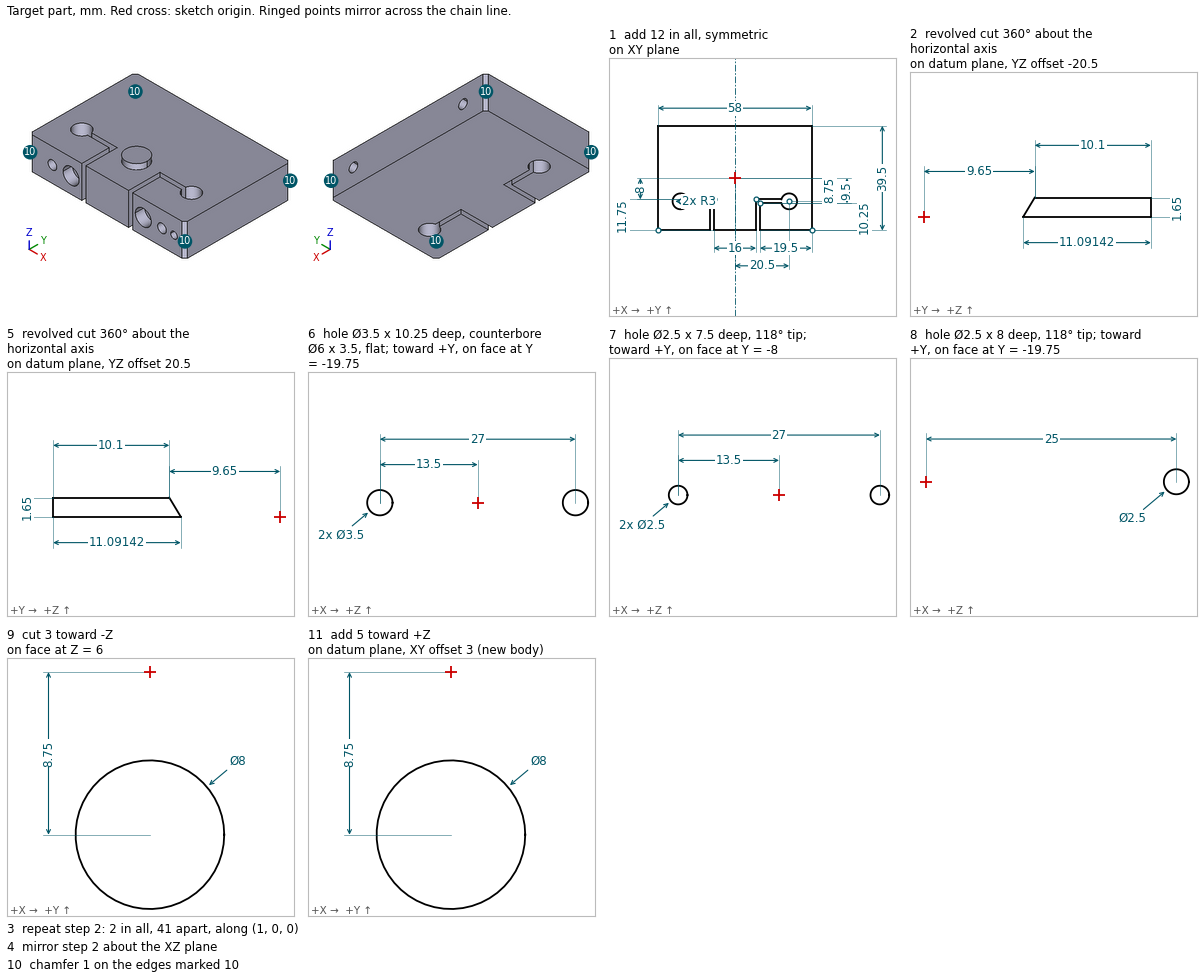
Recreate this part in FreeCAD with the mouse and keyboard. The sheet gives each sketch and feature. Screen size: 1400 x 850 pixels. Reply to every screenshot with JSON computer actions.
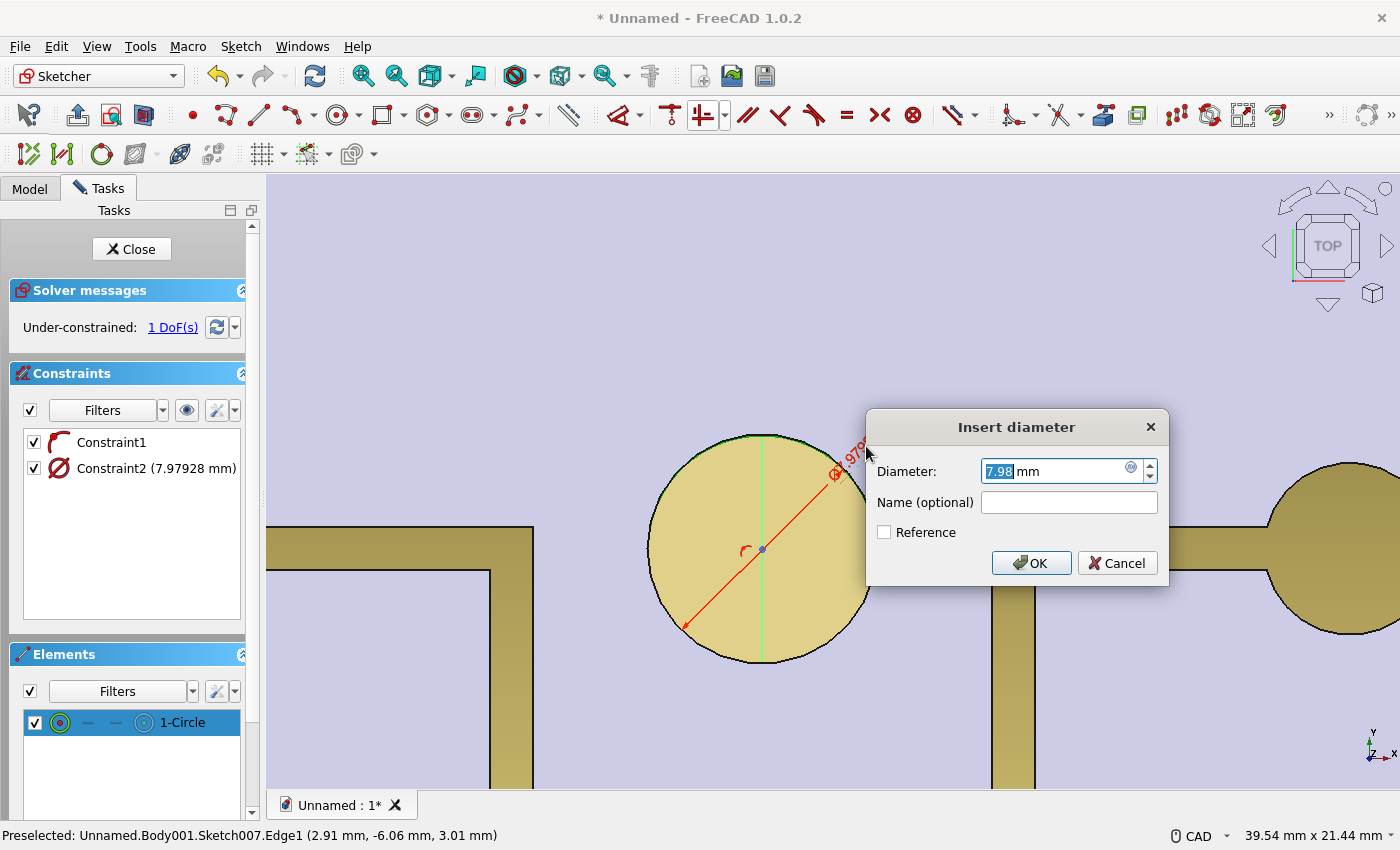
{"action": "type", "text": "8"}
{"action": "key", "text": "Return"}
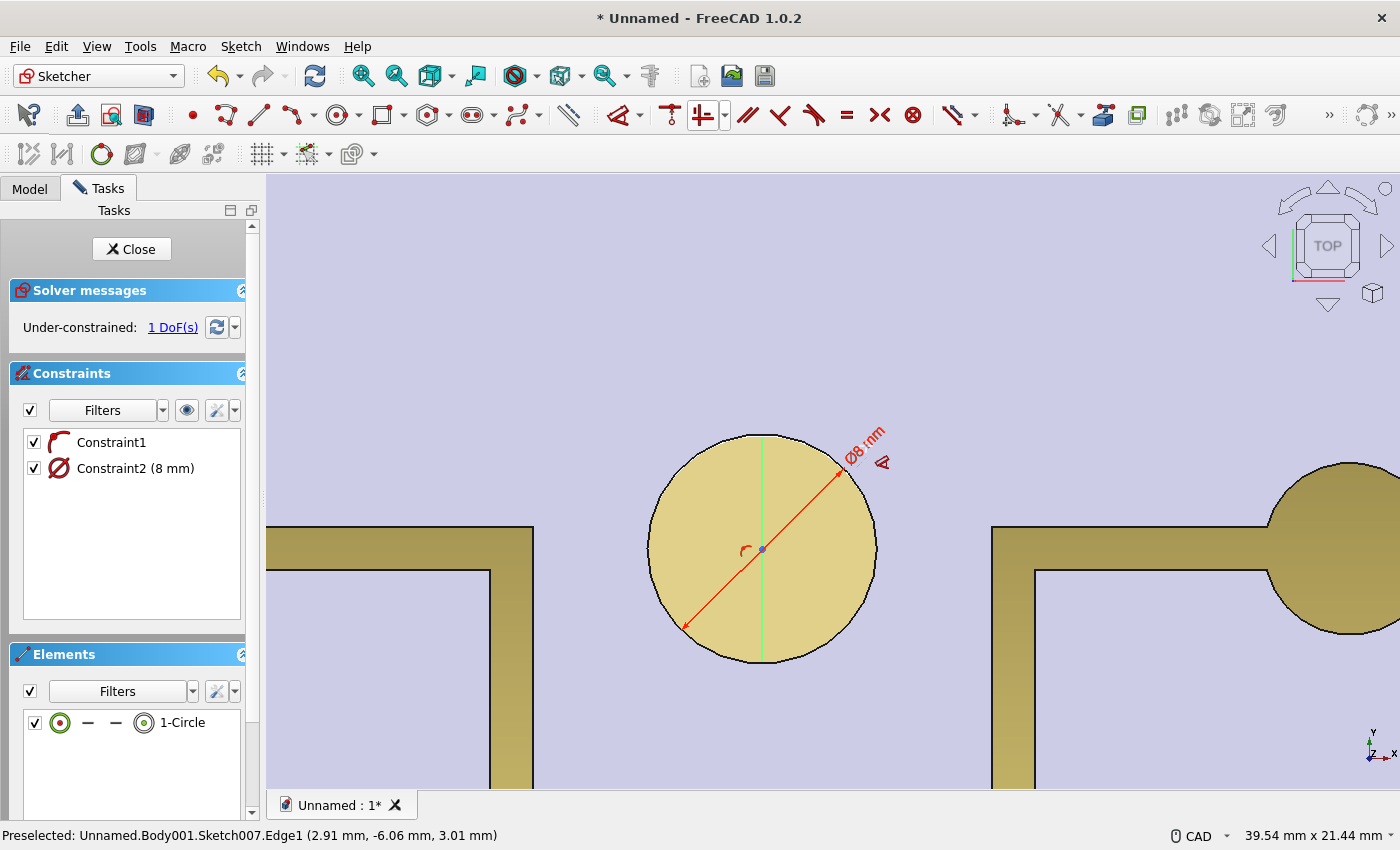
{"action": "left_click", "coordinate": [762, 550]}
{"action": "left_click", "coordinate": [796, 424]}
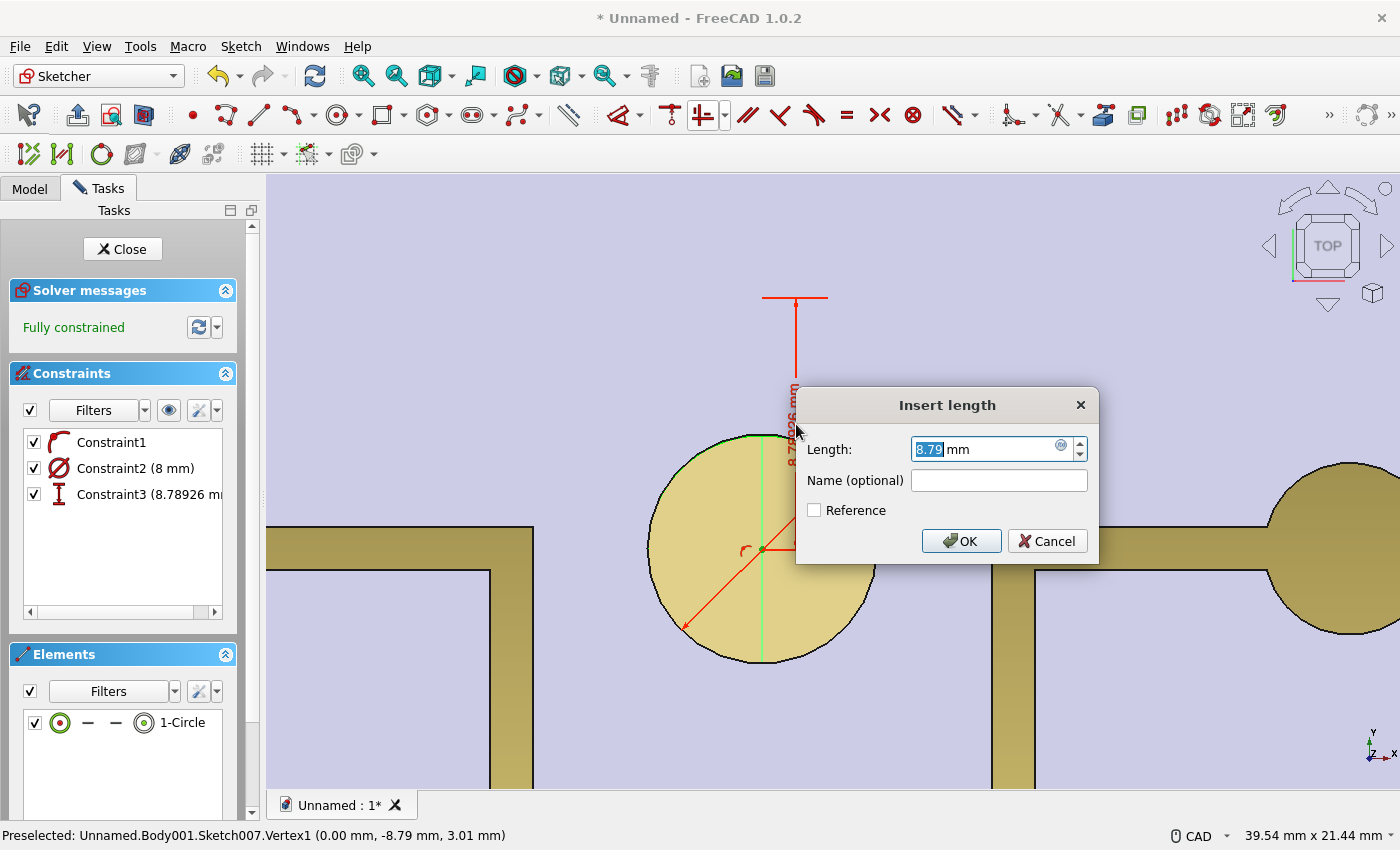
{"action": "type", "text": "8.75"}
{"action": "key", "text": "Return"}
{"action": "key", "text": "Escape"}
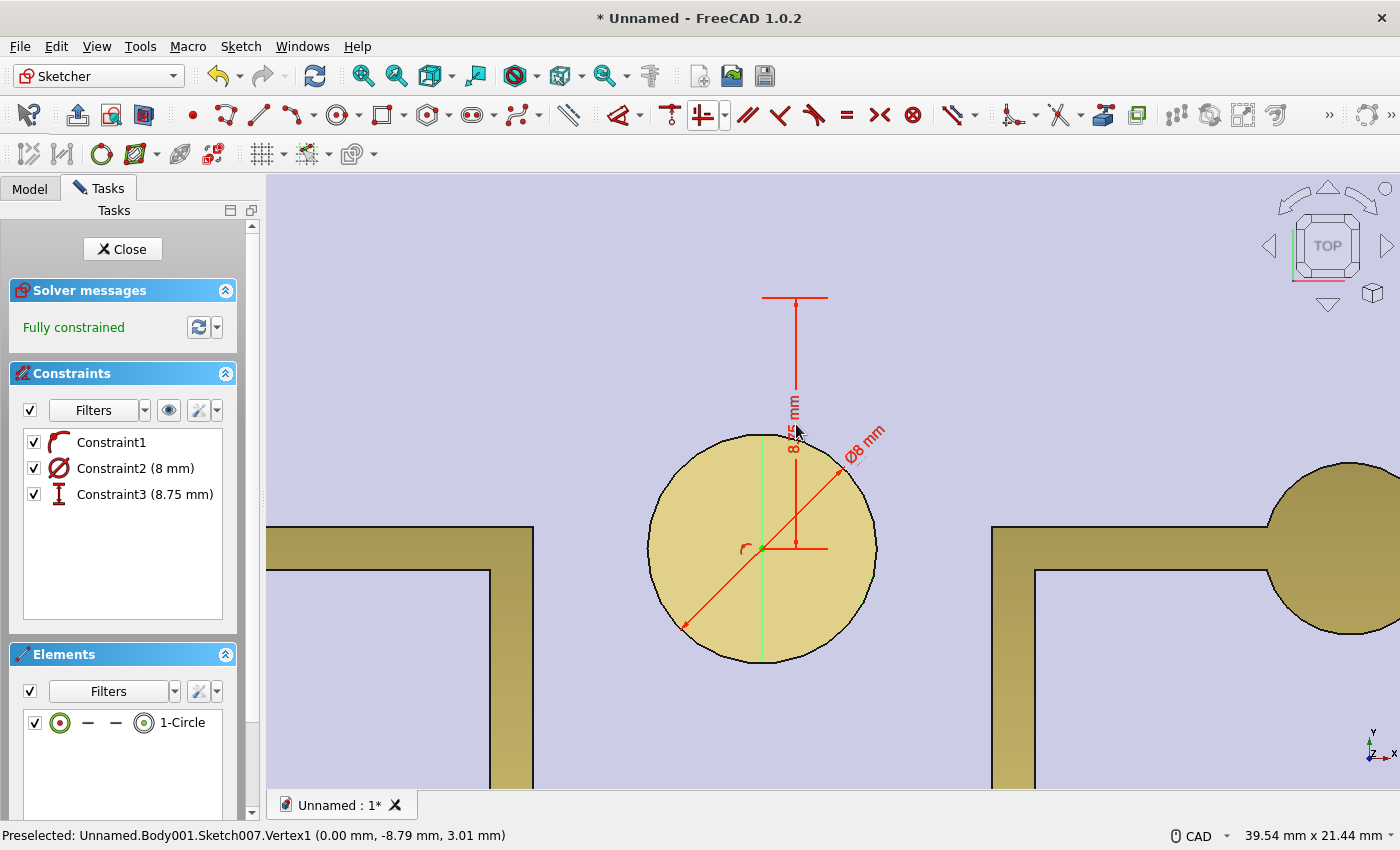
{"action": "left_click", "coordinate": [123, 249]}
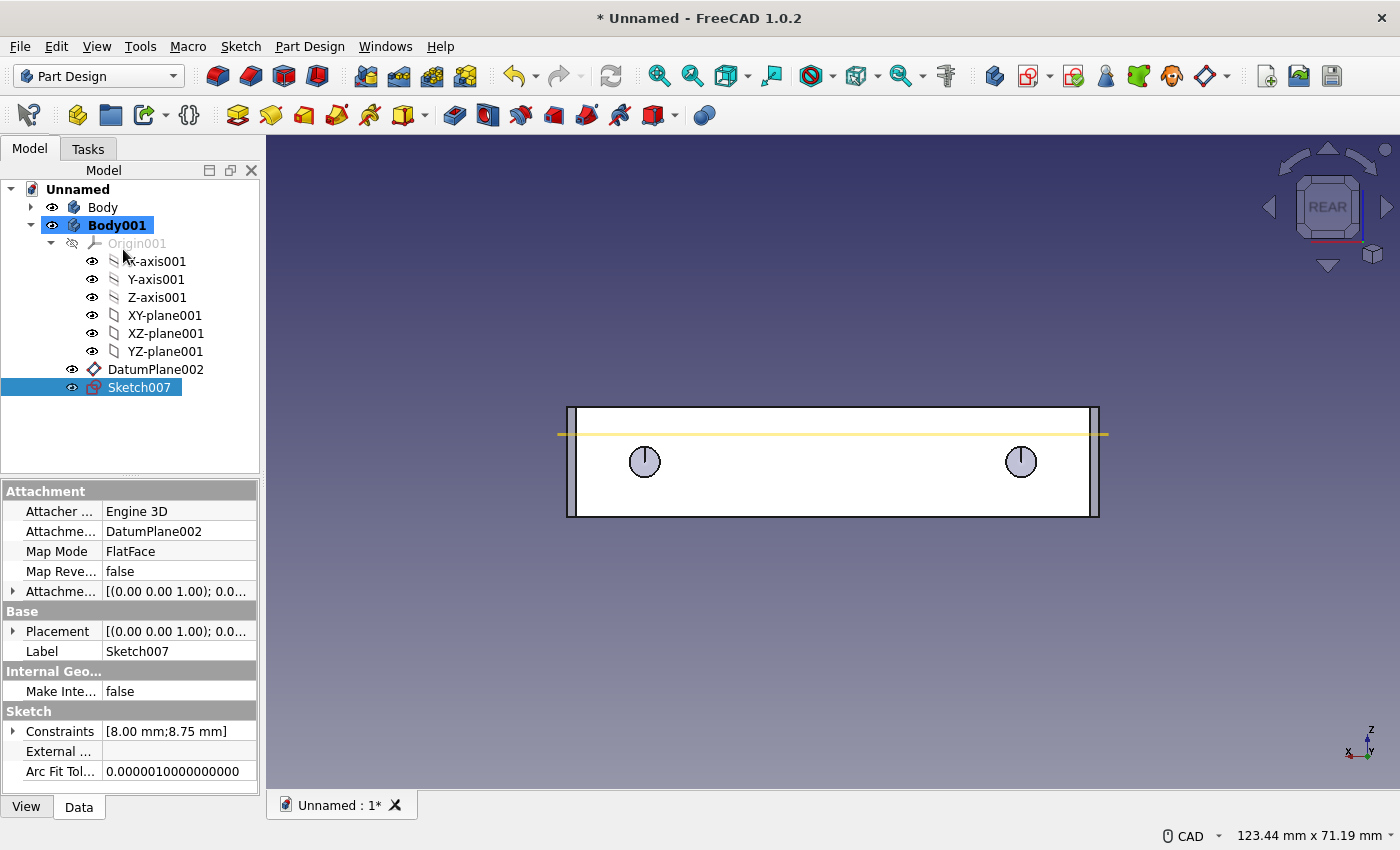
{"action": "left_click", "coordinate": [238, 116]}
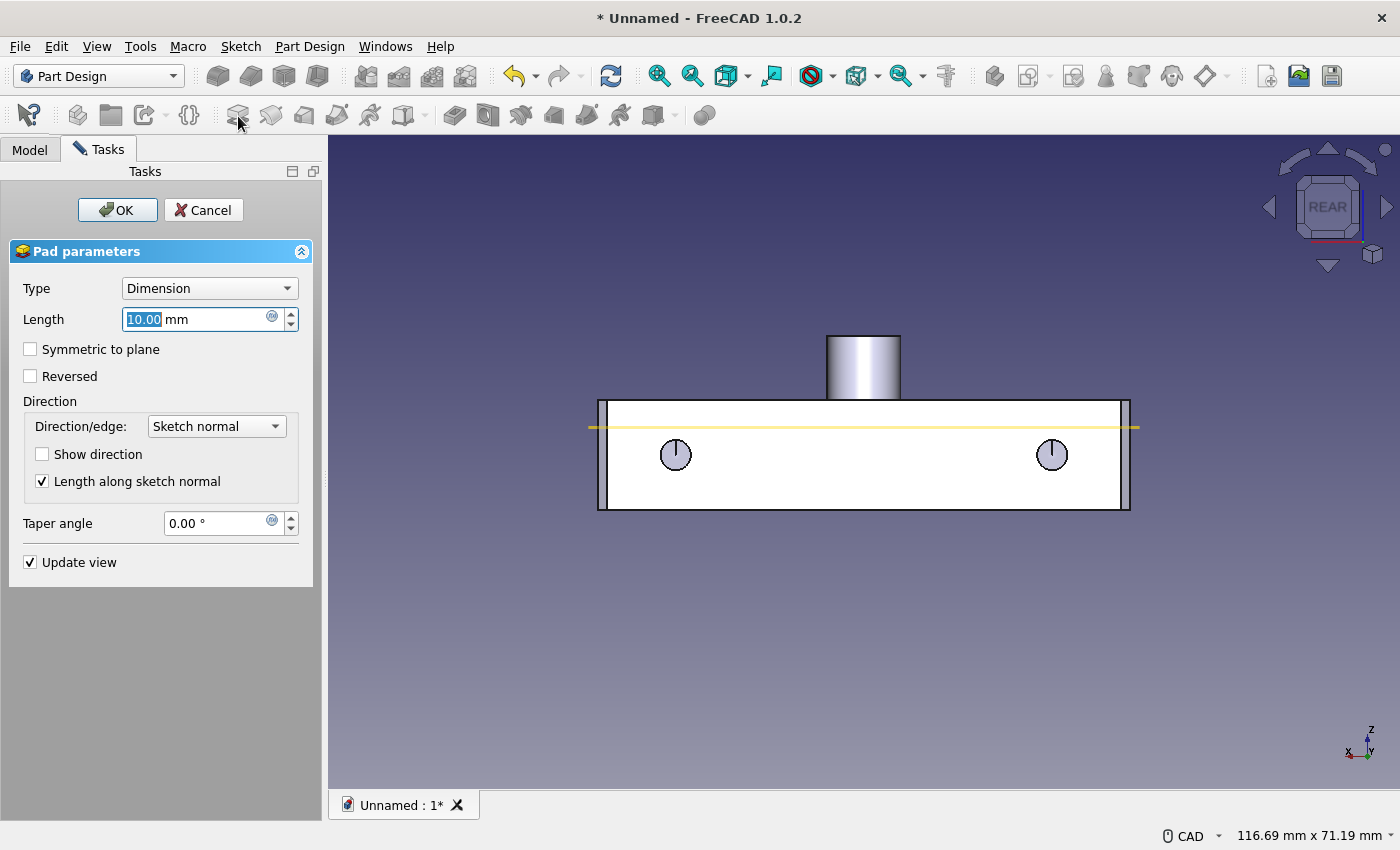
{"action": "type", "text": "5"}
{"action": "key", "text": "Tab"}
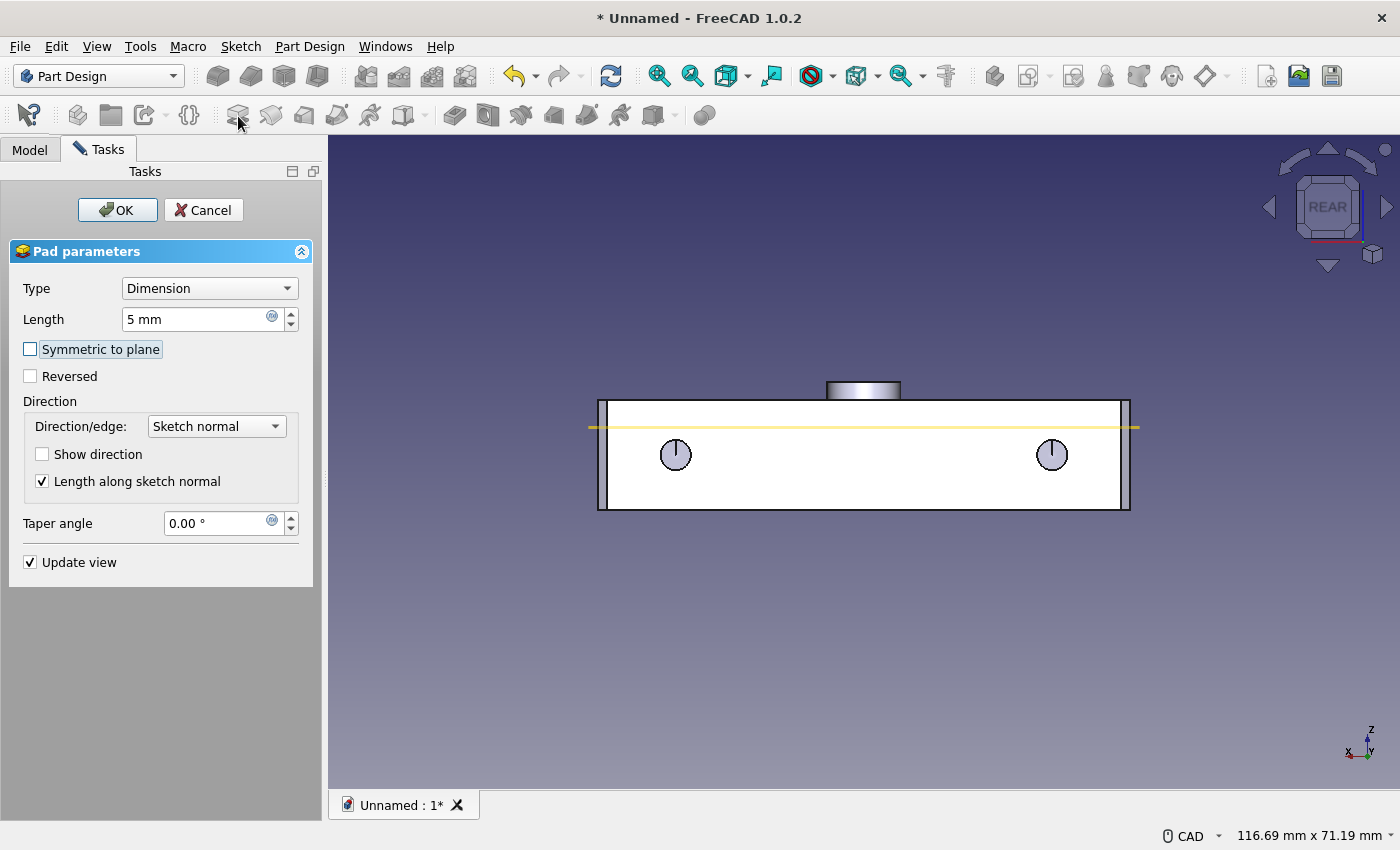
{"action": "left_click", "coordinate": [118, 210]}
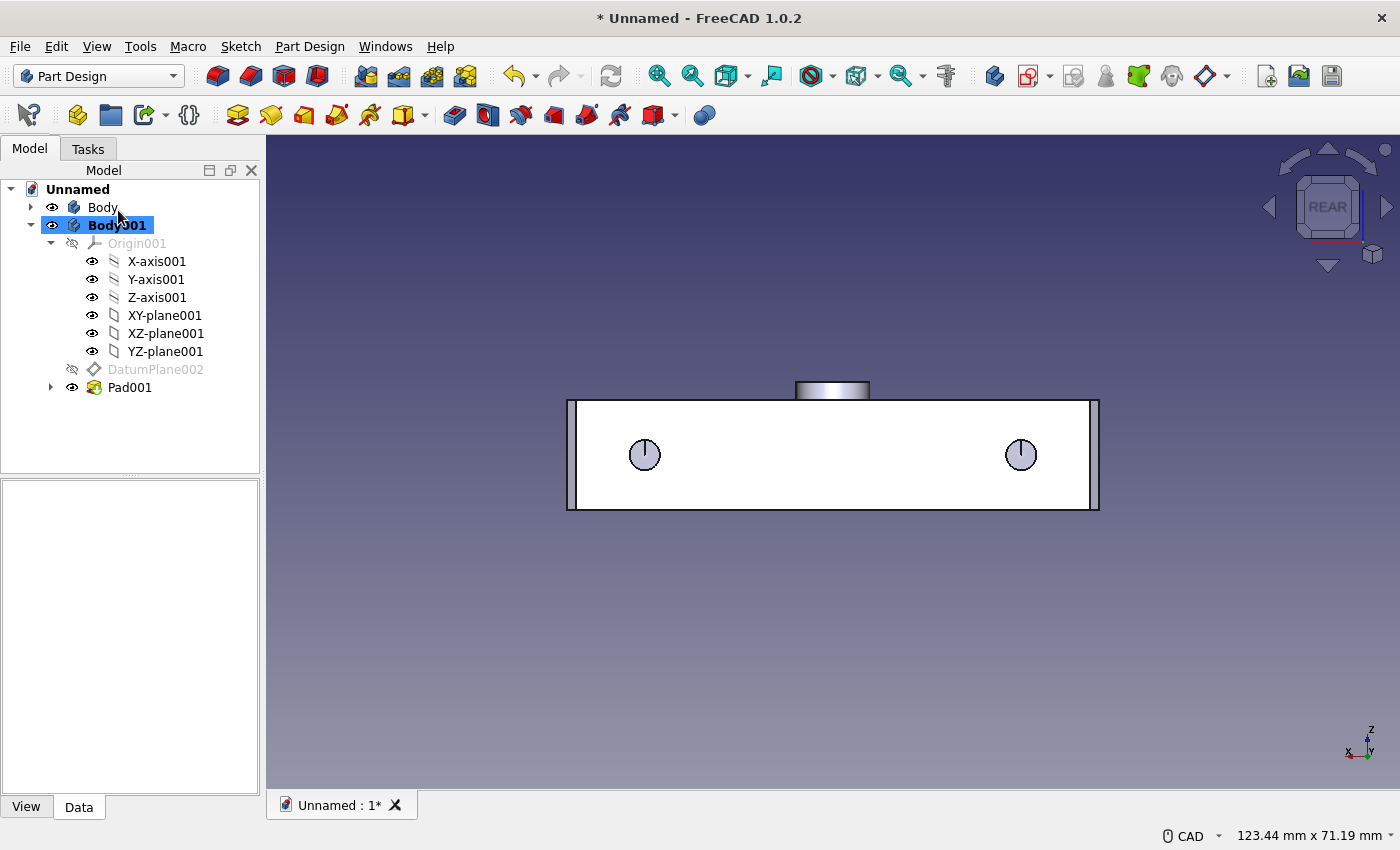
{"action": "key", "text": "0"}